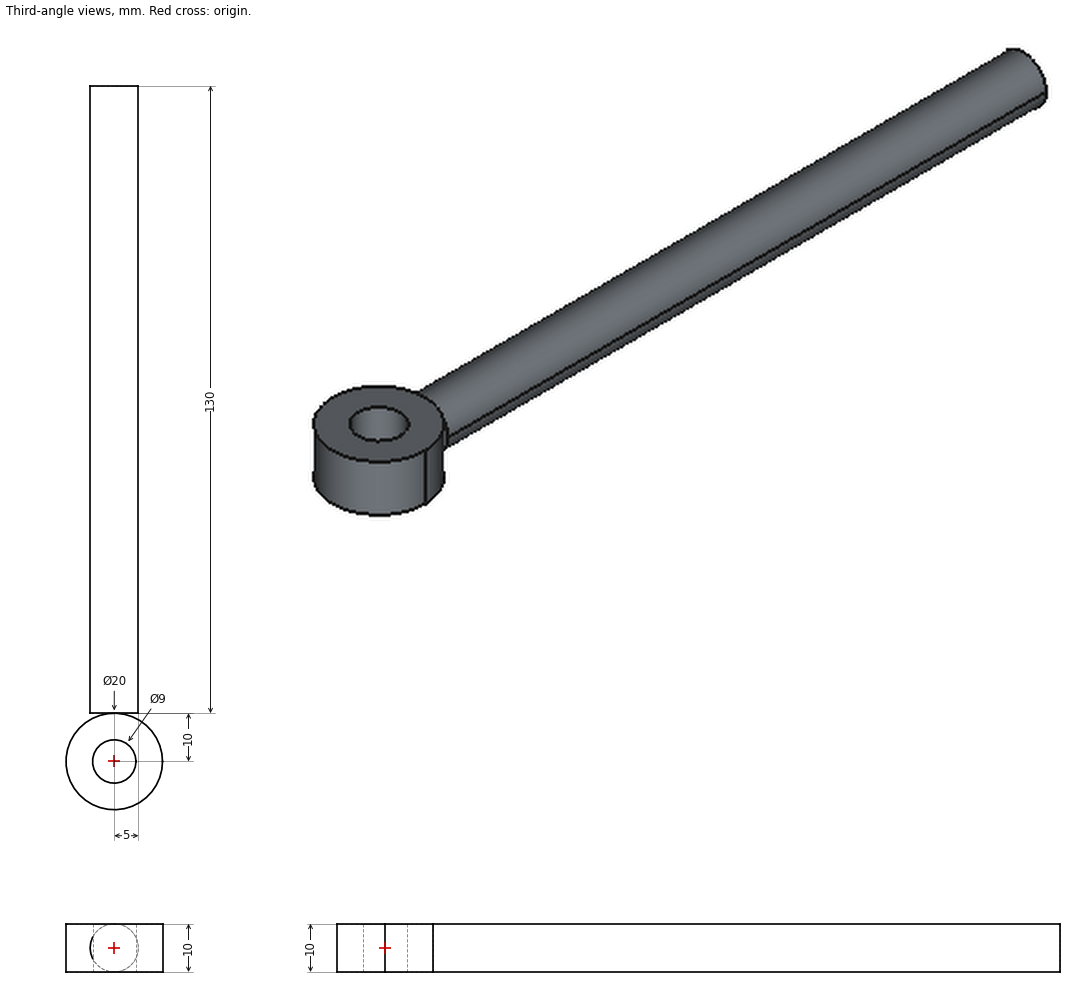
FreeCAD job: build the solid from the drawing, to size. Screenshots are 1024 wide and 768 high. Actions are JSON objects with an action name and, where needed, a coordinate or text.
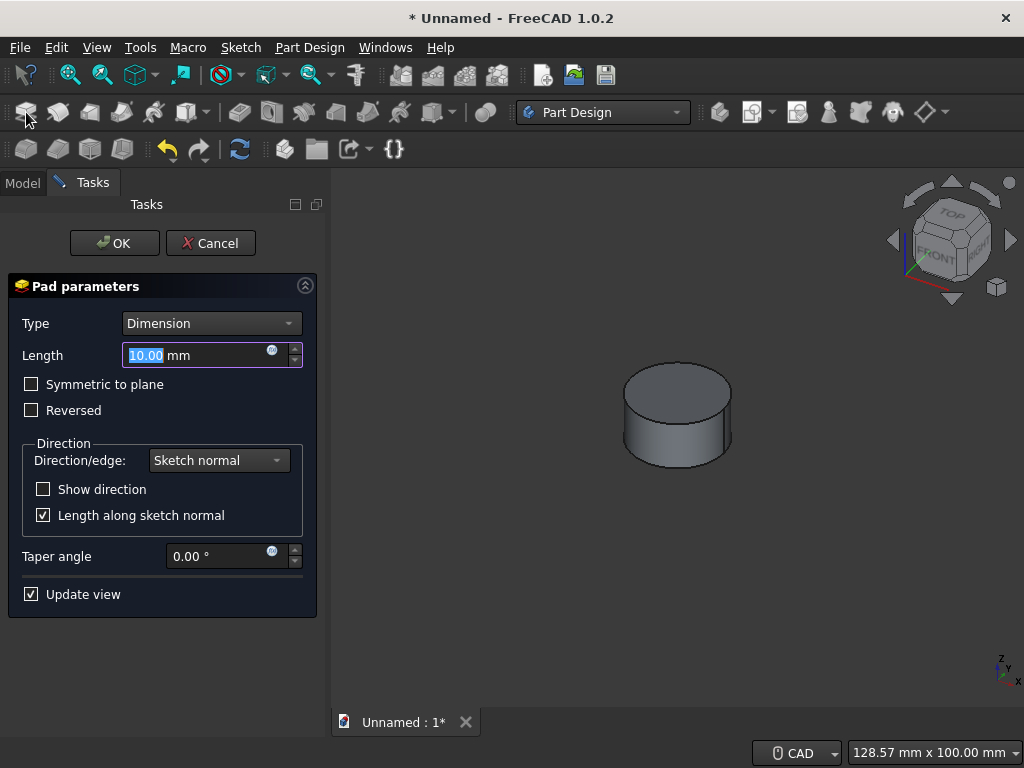
{"action": "type", "text": "10"}
{"action": "key", "text": "Tab"}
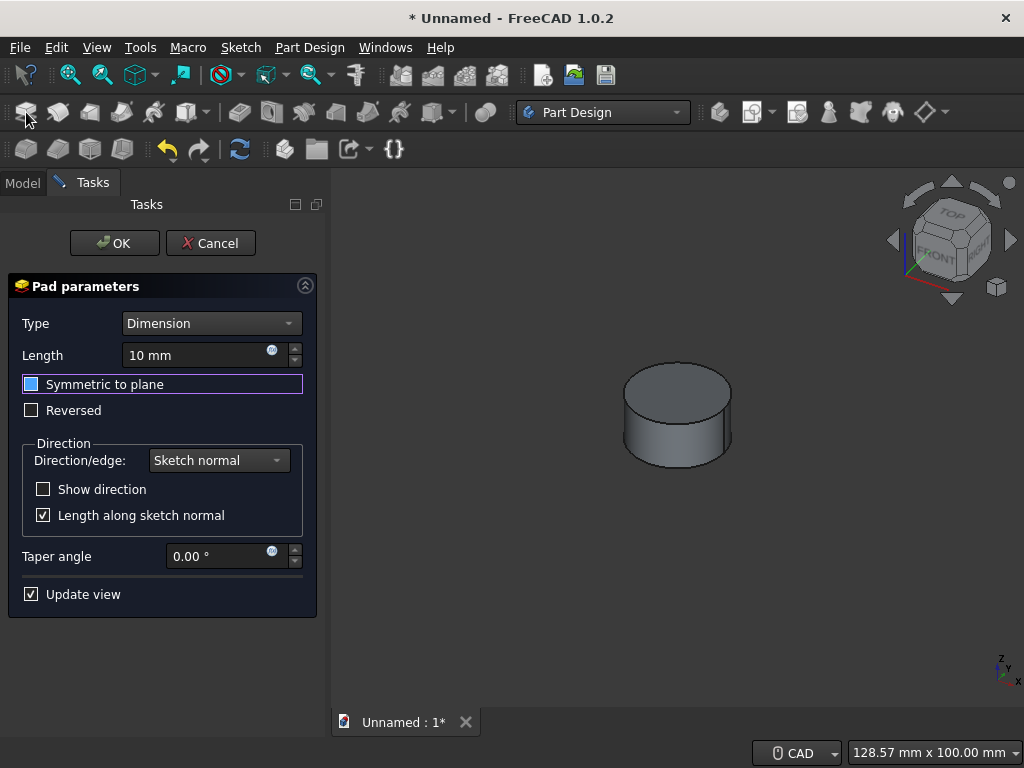
{"action": "left_click", "coordinate": [30, 384]}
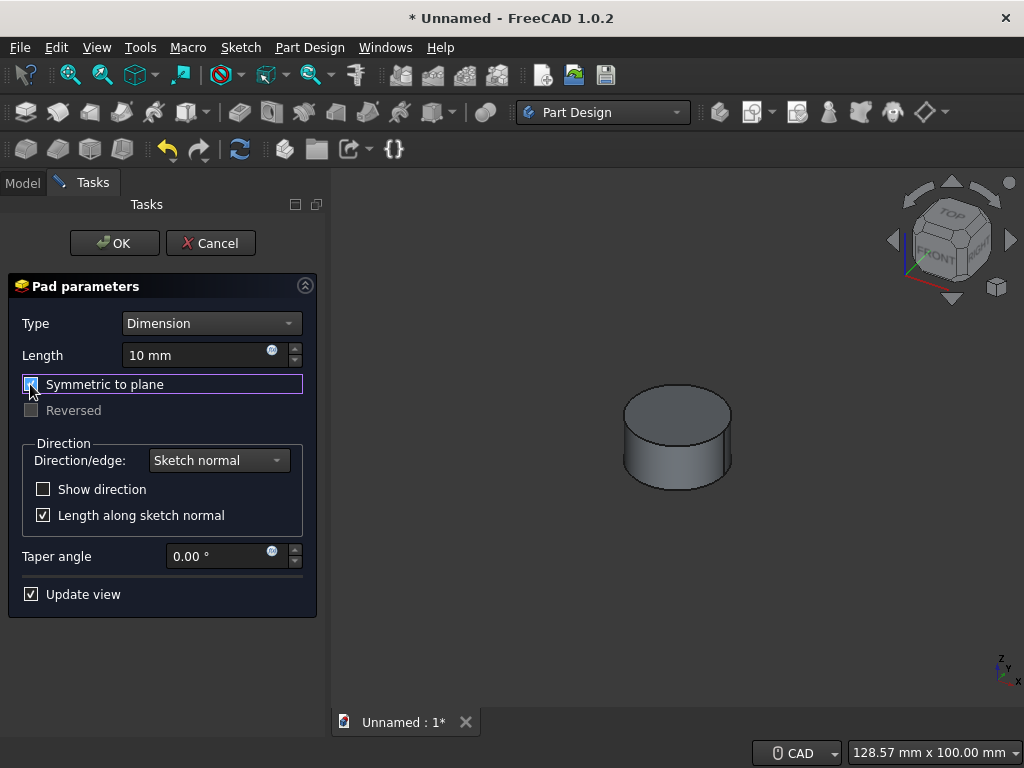
{"action": "left_click", "coordinate": [115, 243]}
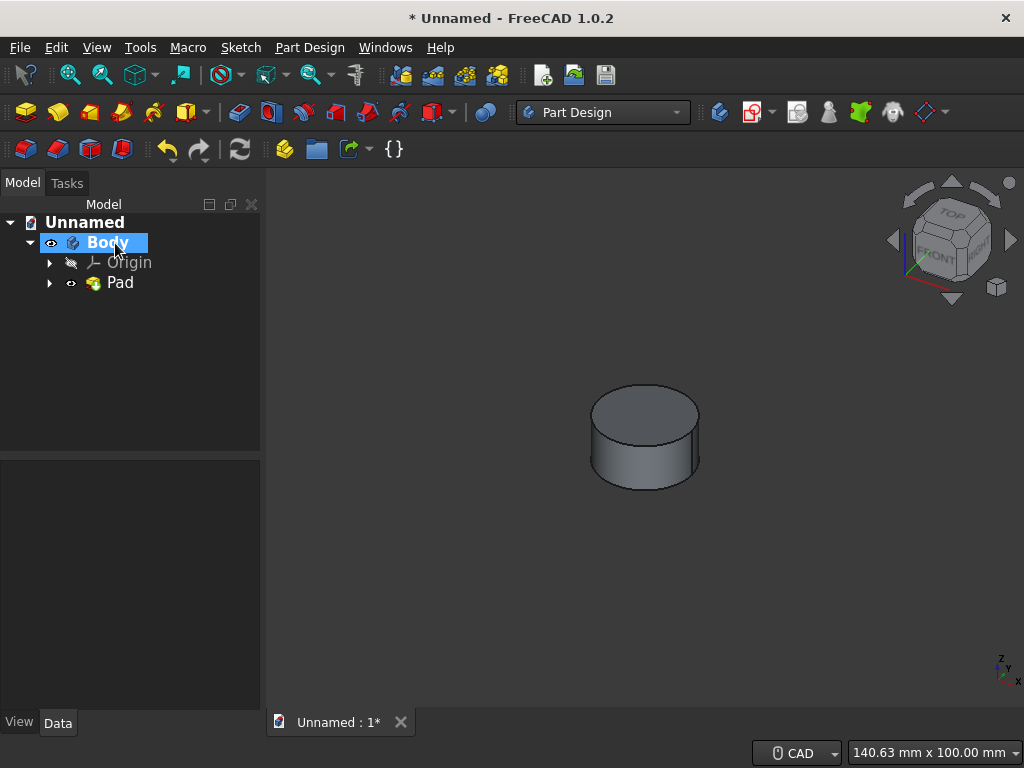
{"action": "left_click", "coordinate": [72, 76]}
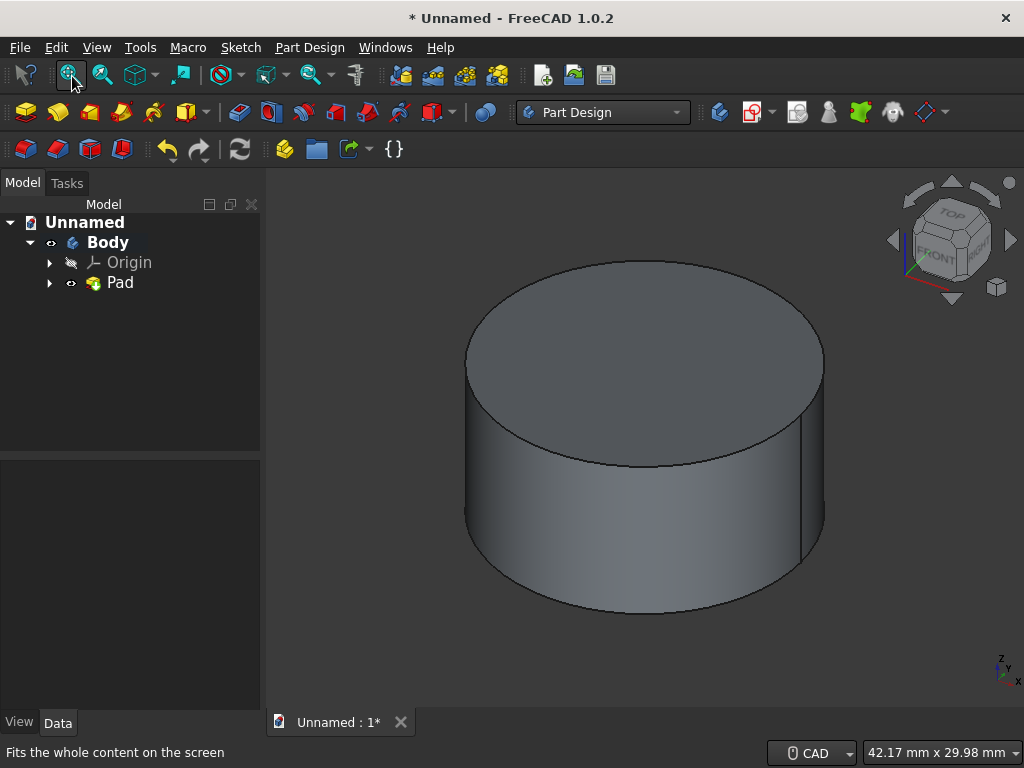
{"action": "left_click", "coordinate": [645, 363]}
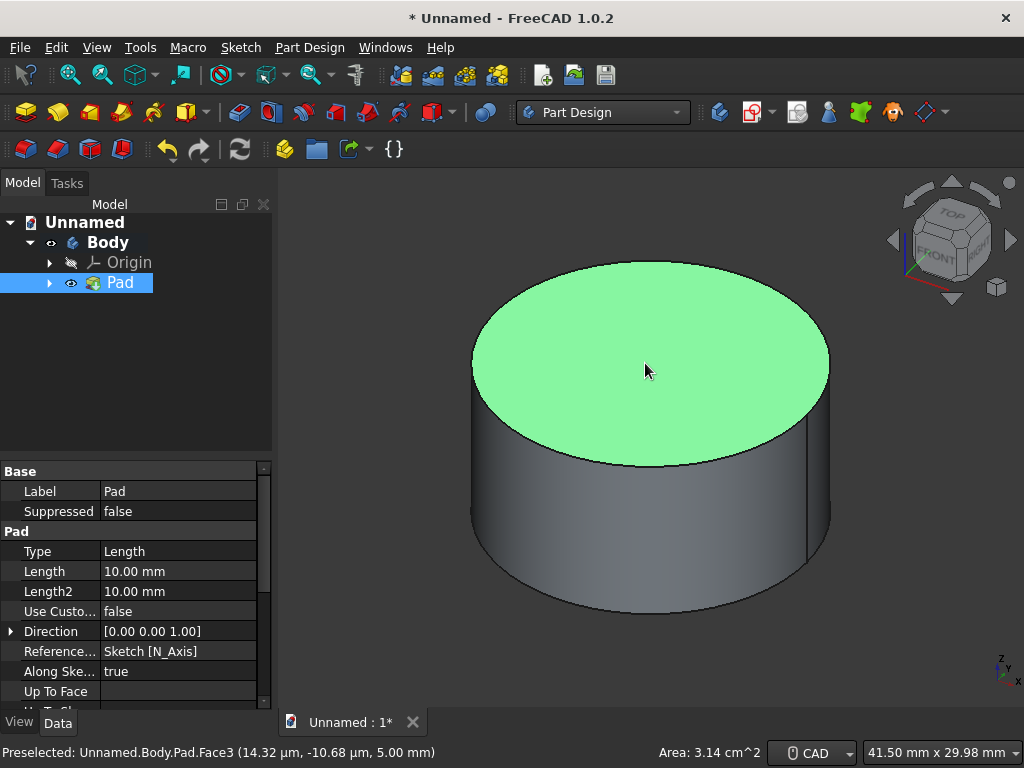
{"action": "left_click", "coordinate": [752, 112]}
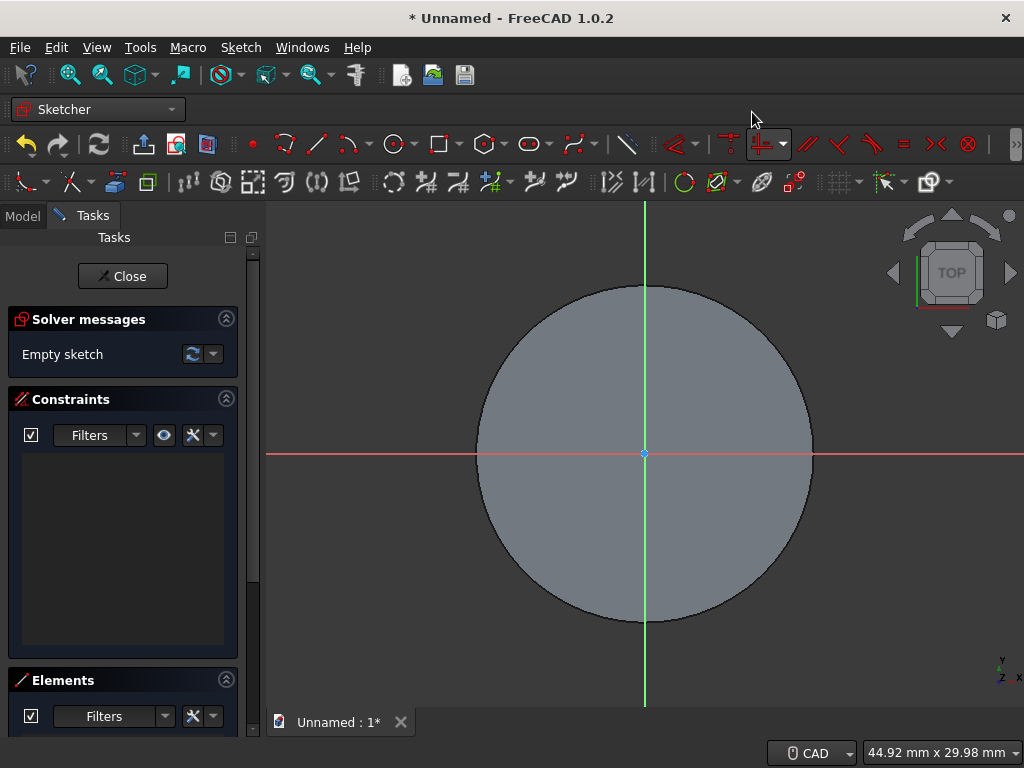
{"action": "scroll", "coordinate": [701, 454], "scroll_direction": "up", "scroll_amount": 4}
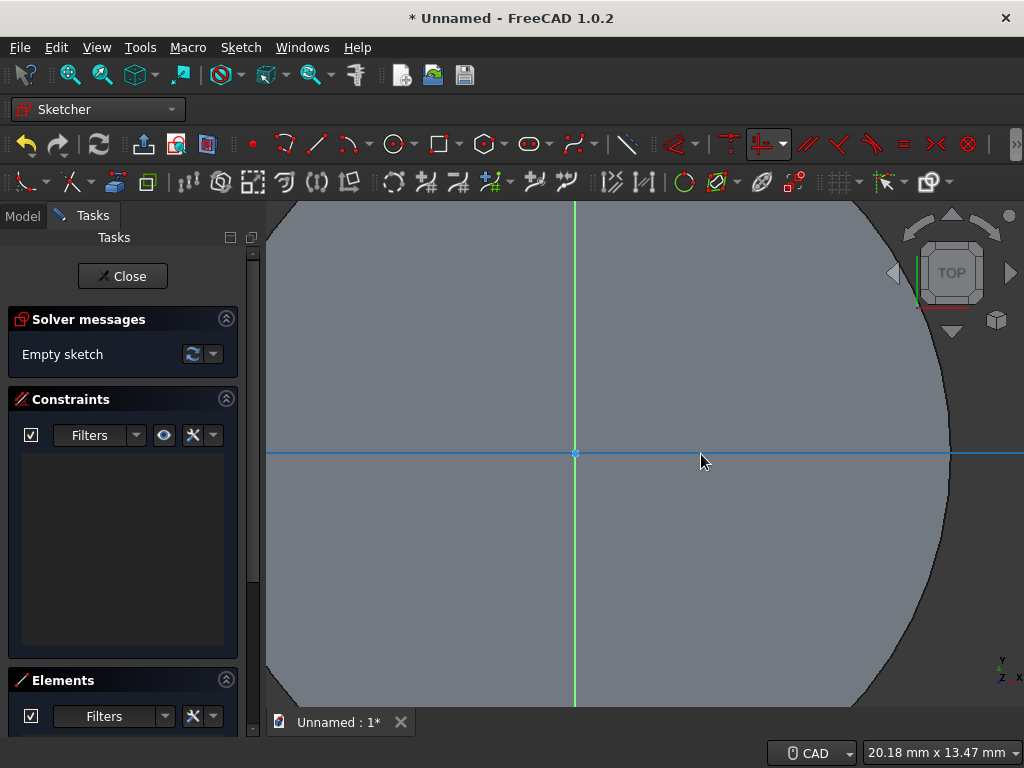
{"action": "left_click", "coordinate": [394, 144]}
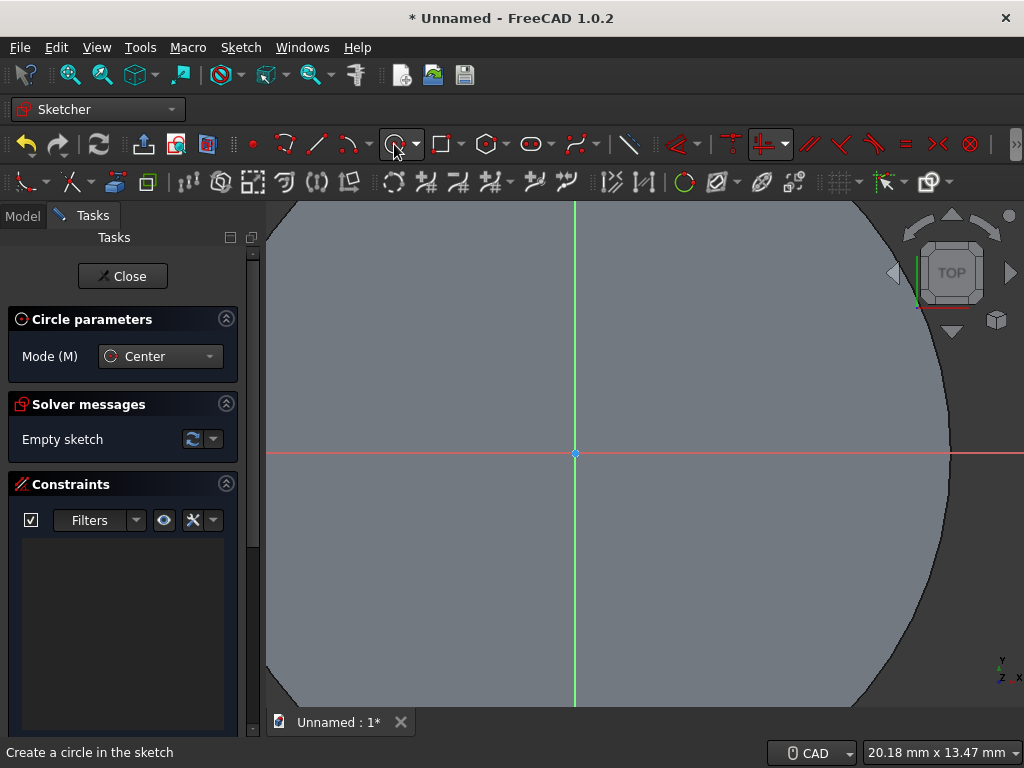
{"action": "left_click", "coordinate": [575, 453]}
{"action": "left_click", "coordinate": [695, 334]}
{"action": "key", "text": "Escape"}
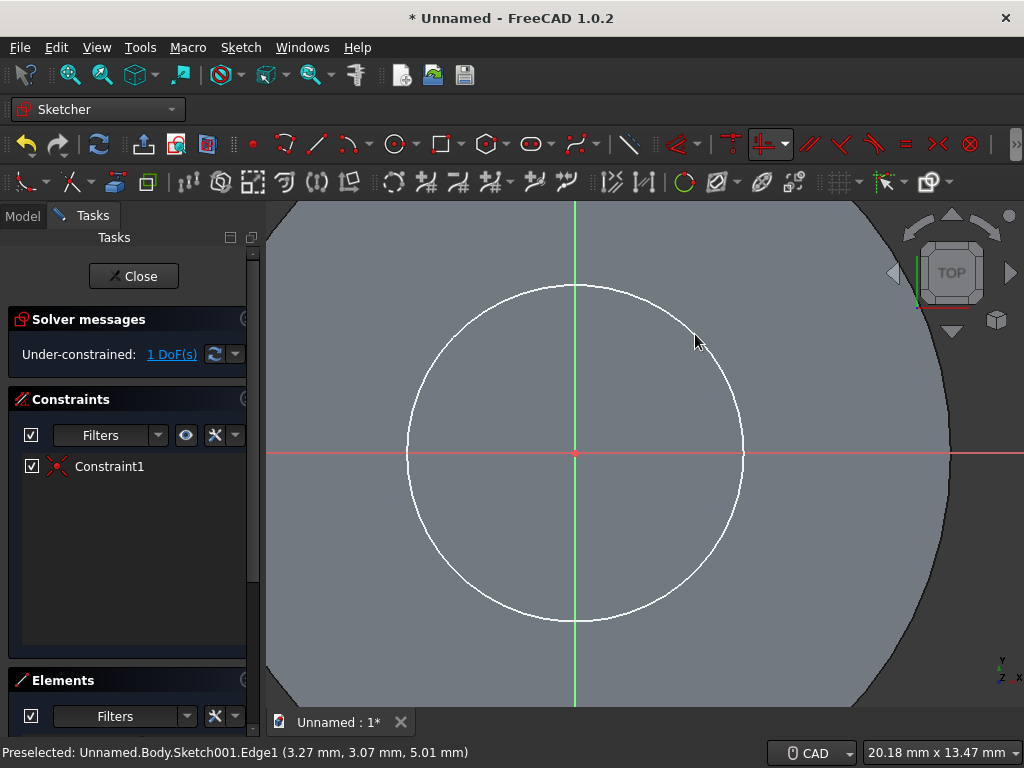
{"action": "left_click", "coordinate": [676, 144]}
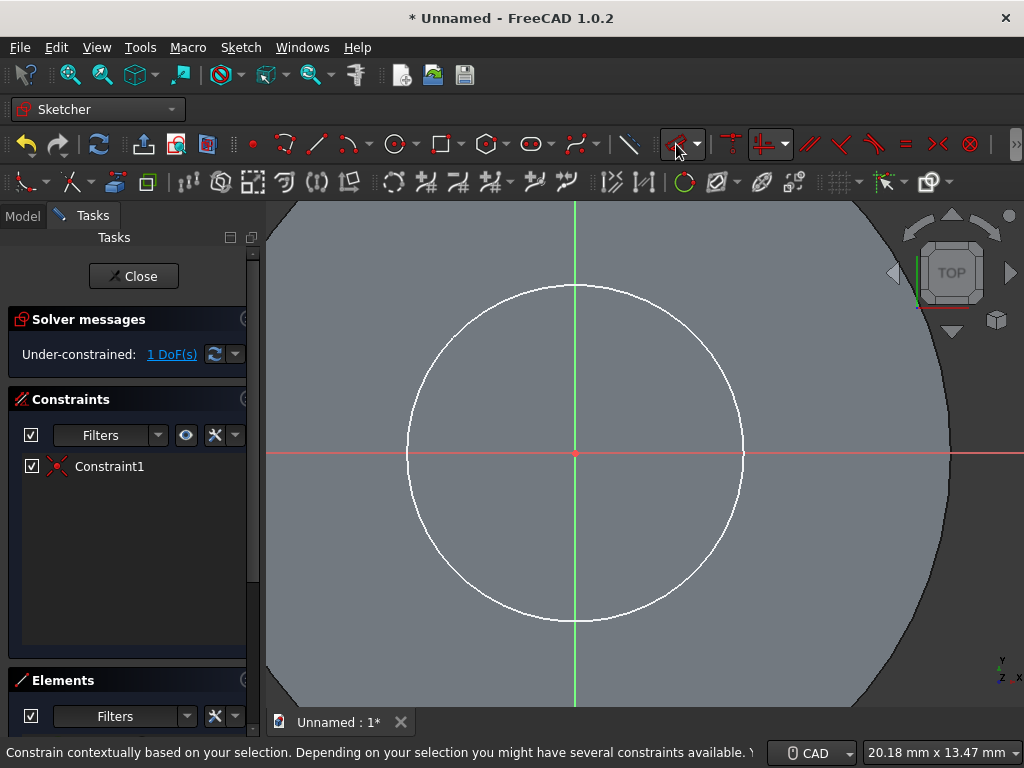
{"action": "left_click", "coordinate": [694, 334]}
{"action": "left_click", "coordinate": [717, 311]}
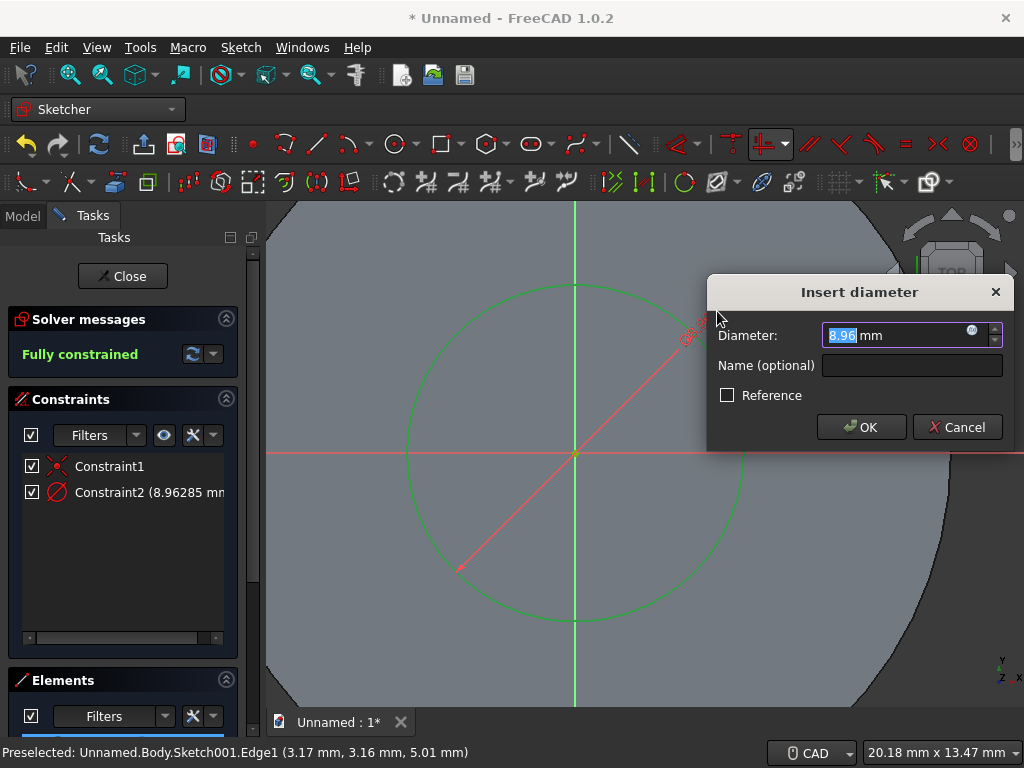
{"action": "type", "text": "9"}
{"action": "key", "text": "Return"}
{"action": "key", "text": "Escape"}